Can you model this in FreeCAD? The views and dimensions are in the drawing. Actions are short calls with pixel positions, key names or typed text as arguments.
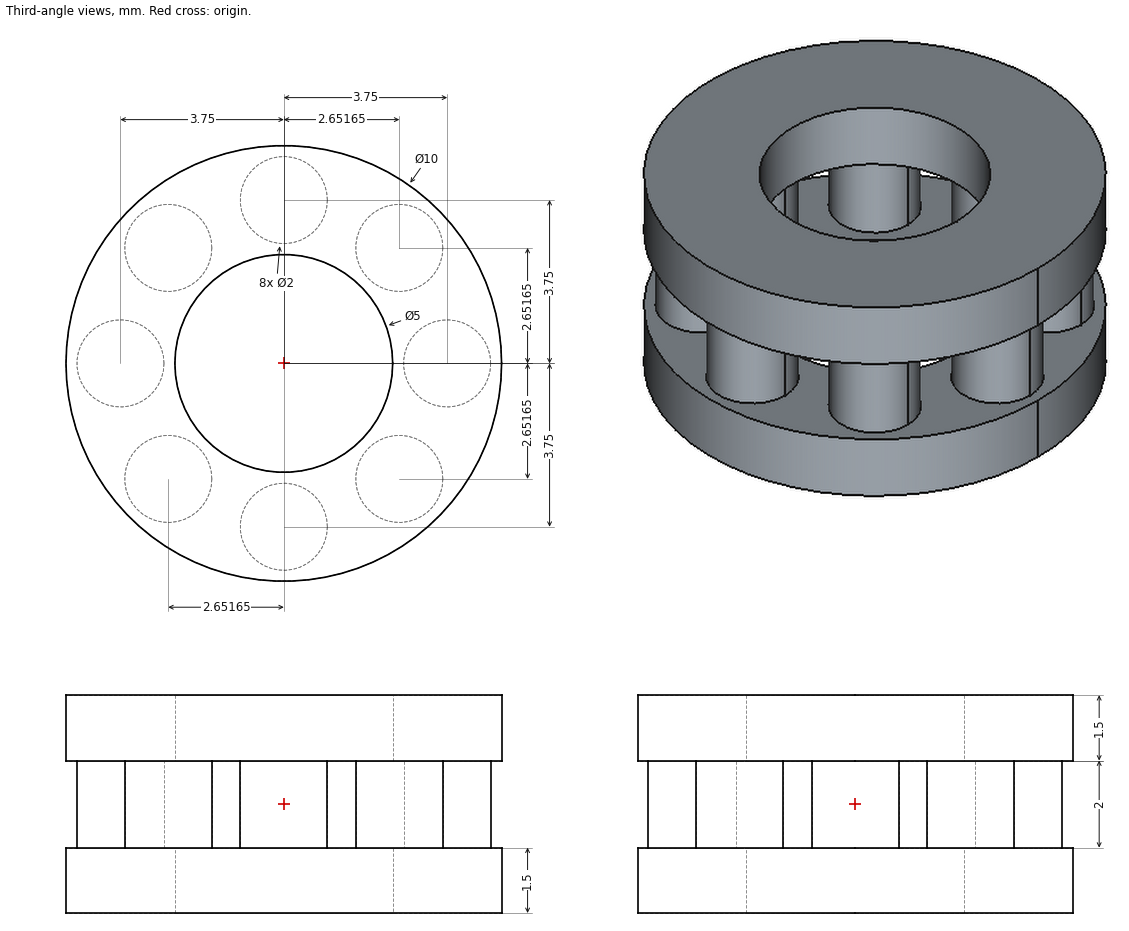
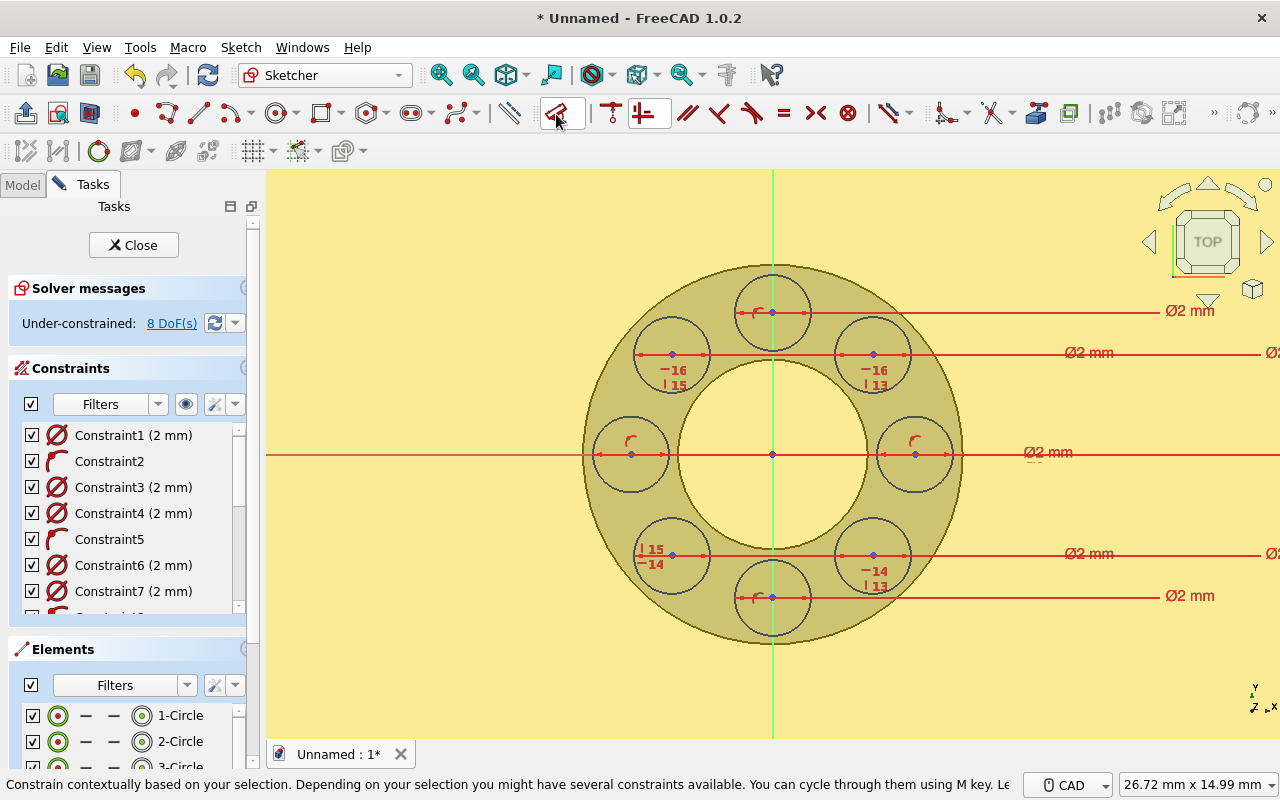
click(773, 313)
click(807, 384)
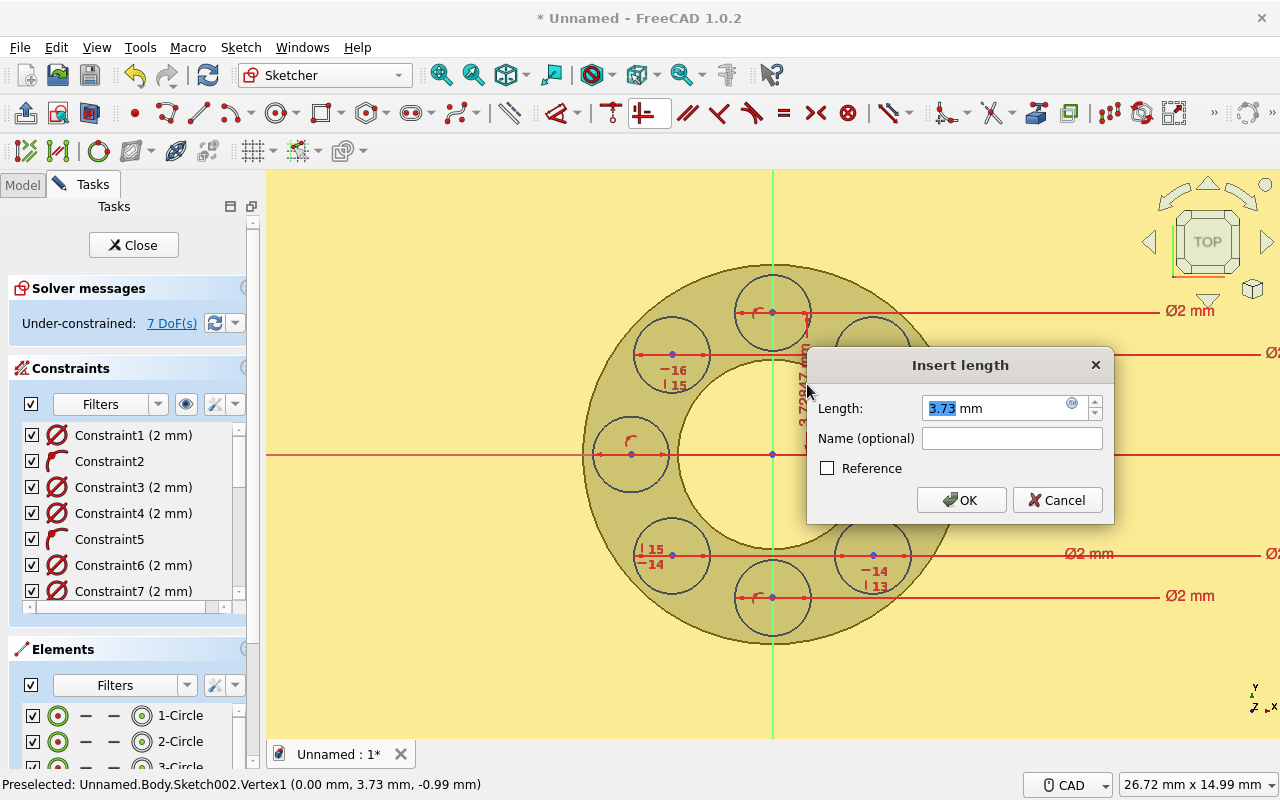
text(3.75)
key(Return)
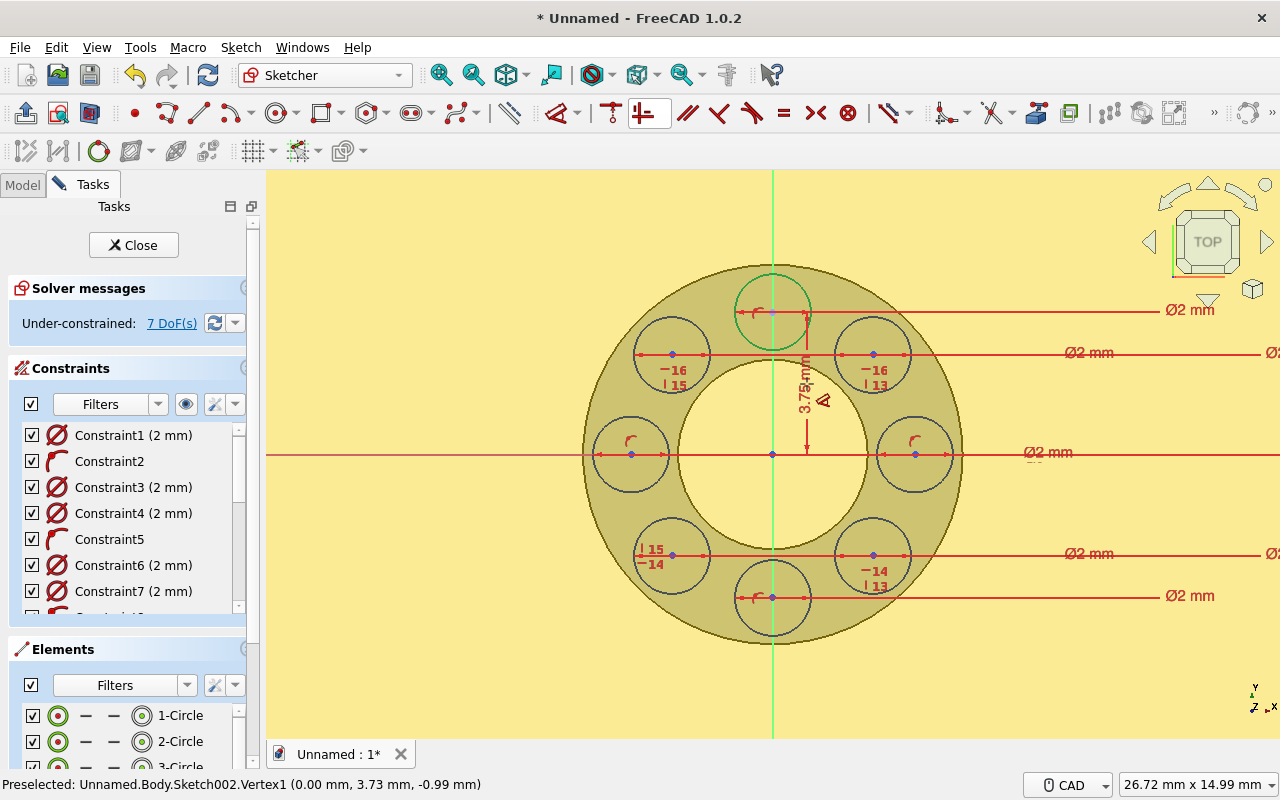
click(915, 454)
click(844, 488)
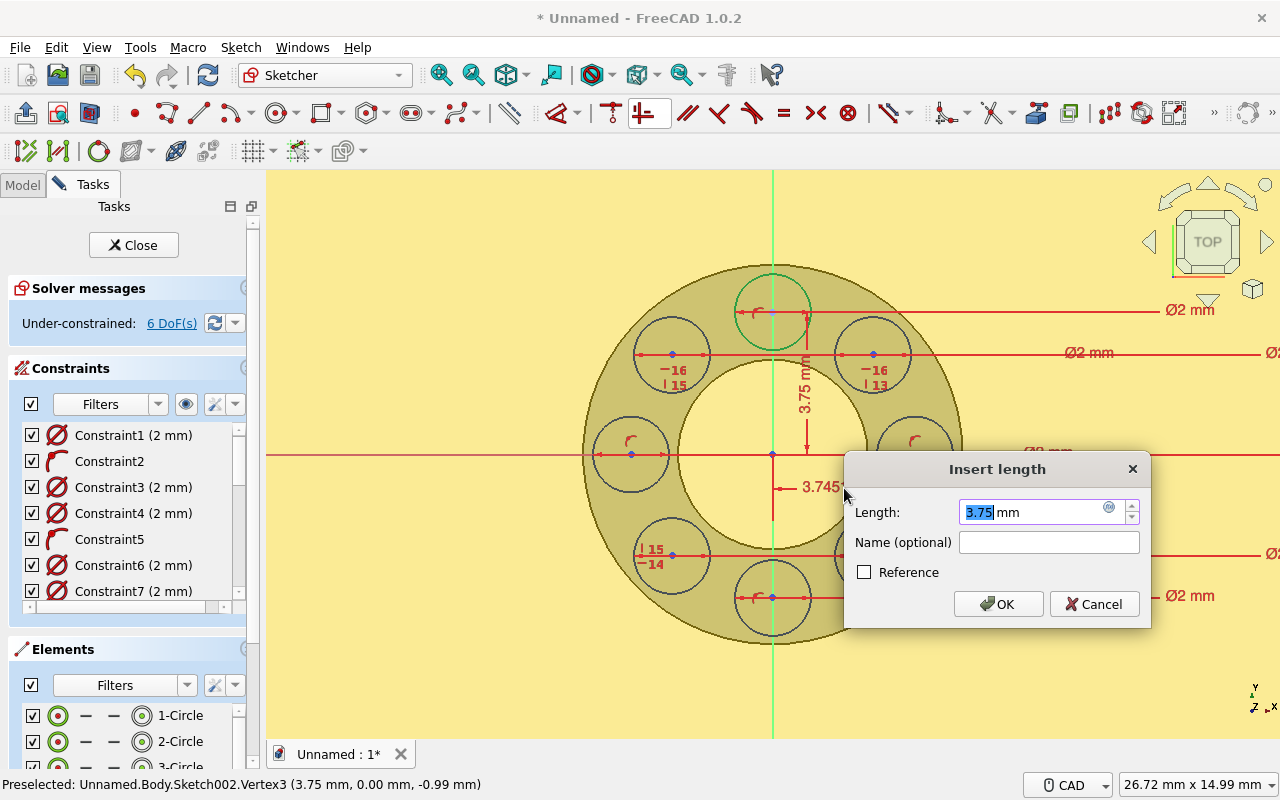
text(3.75)
key(Return)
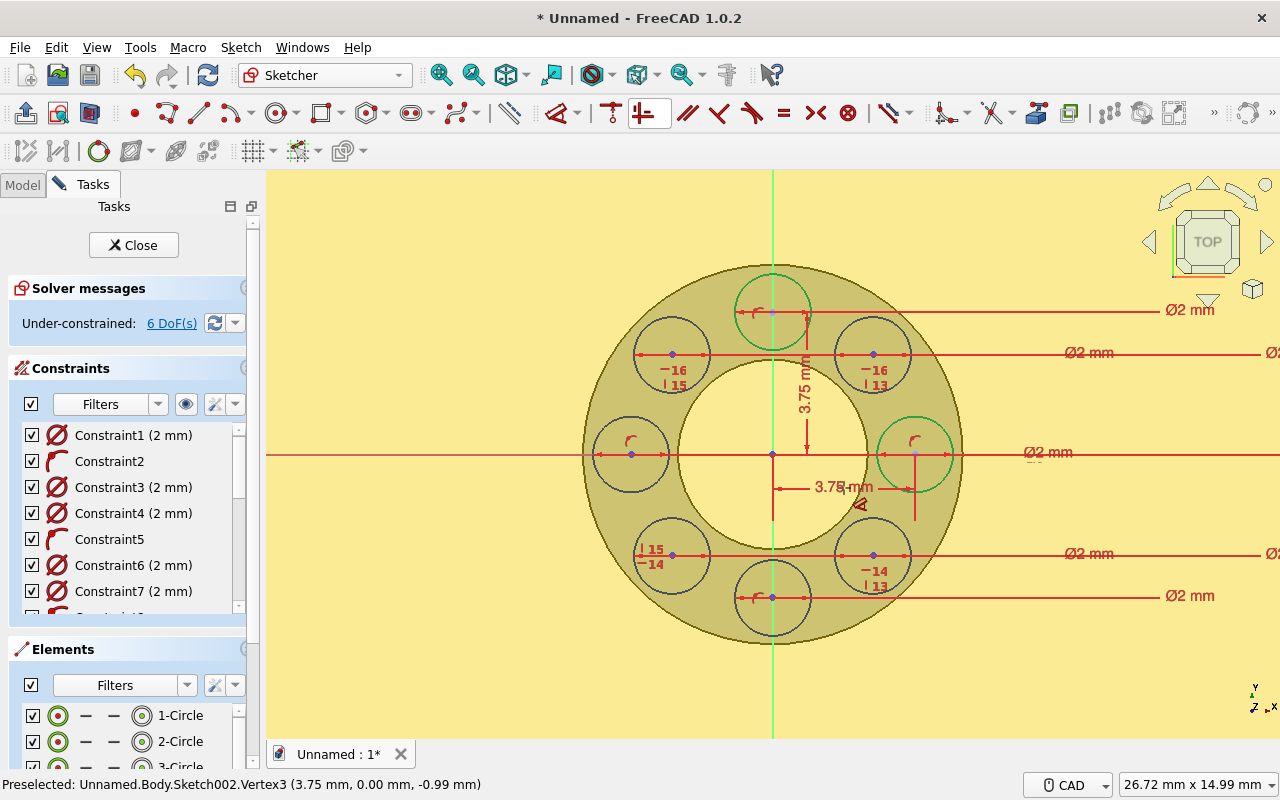
click(773, 598)
click(807, 526)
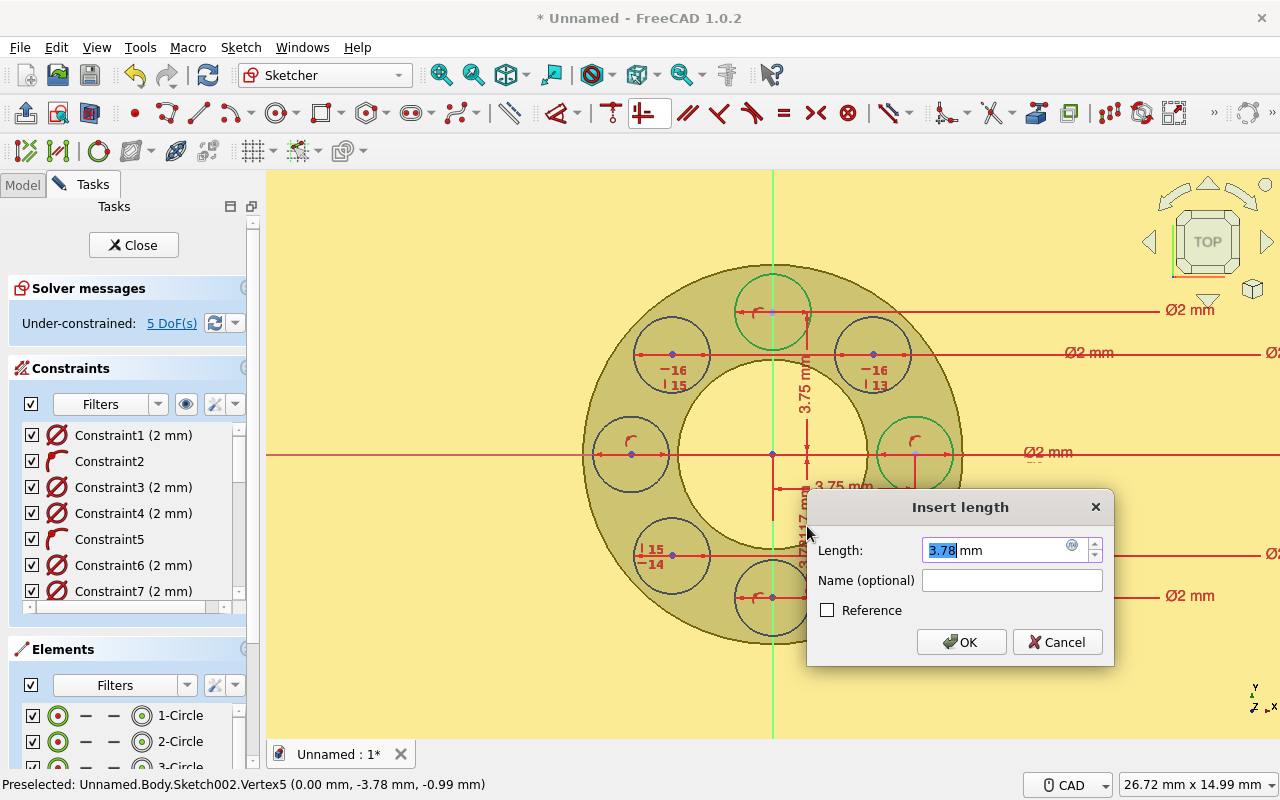
text(3.75)
key(Return)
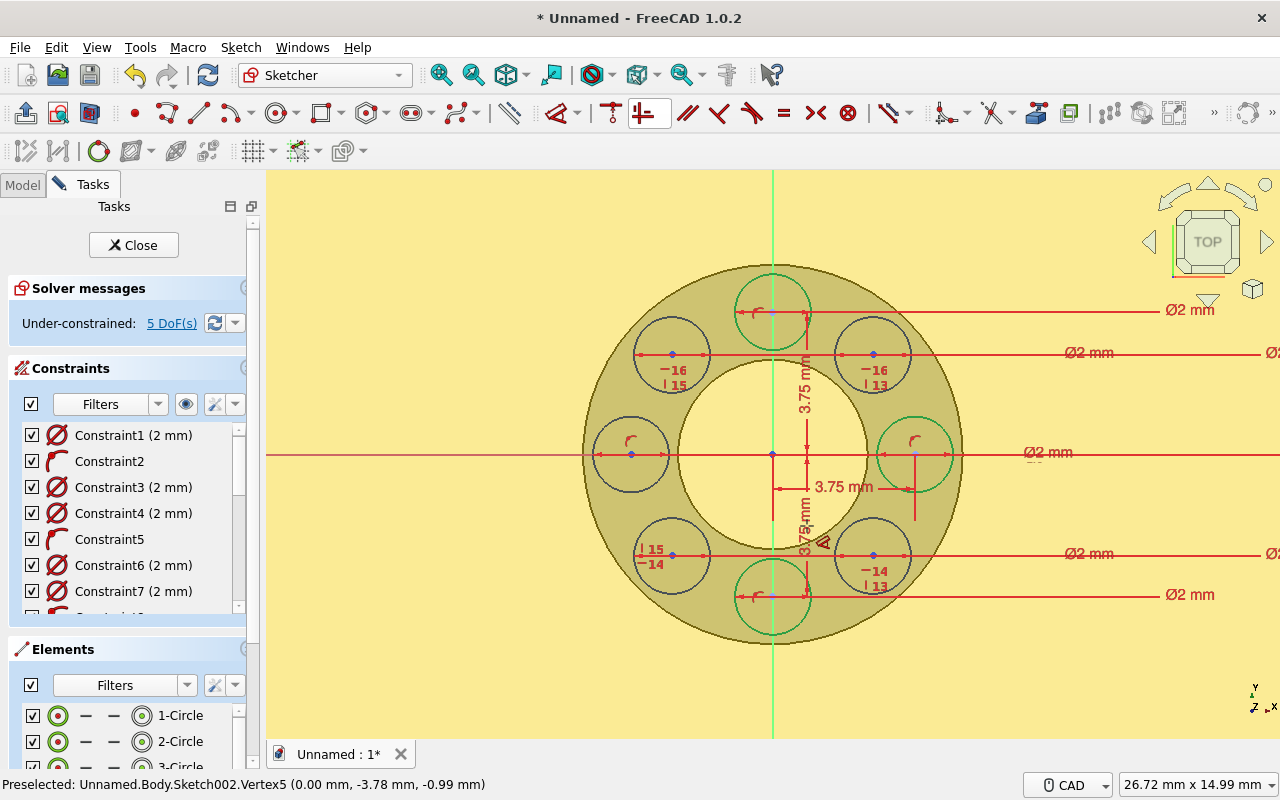
click(631, 454)
click(702, 488)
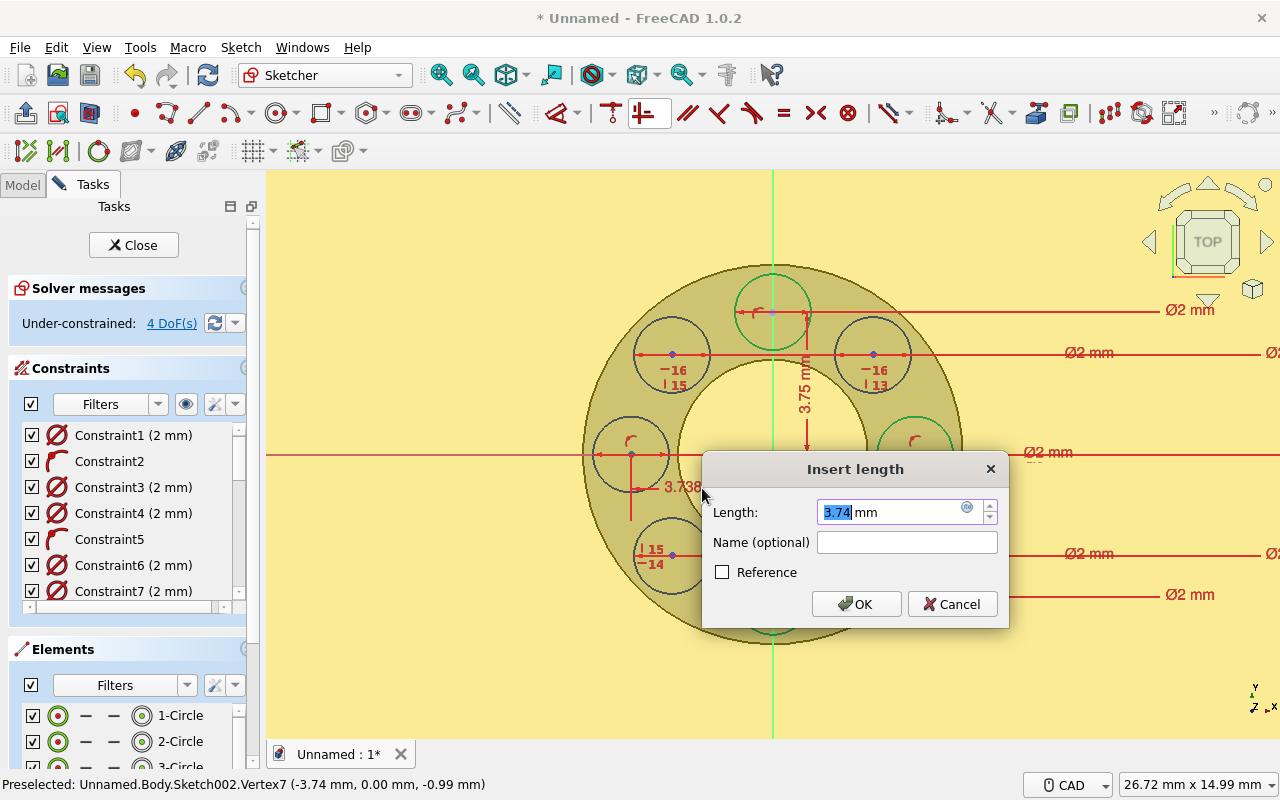
text(3.75)
key(Return)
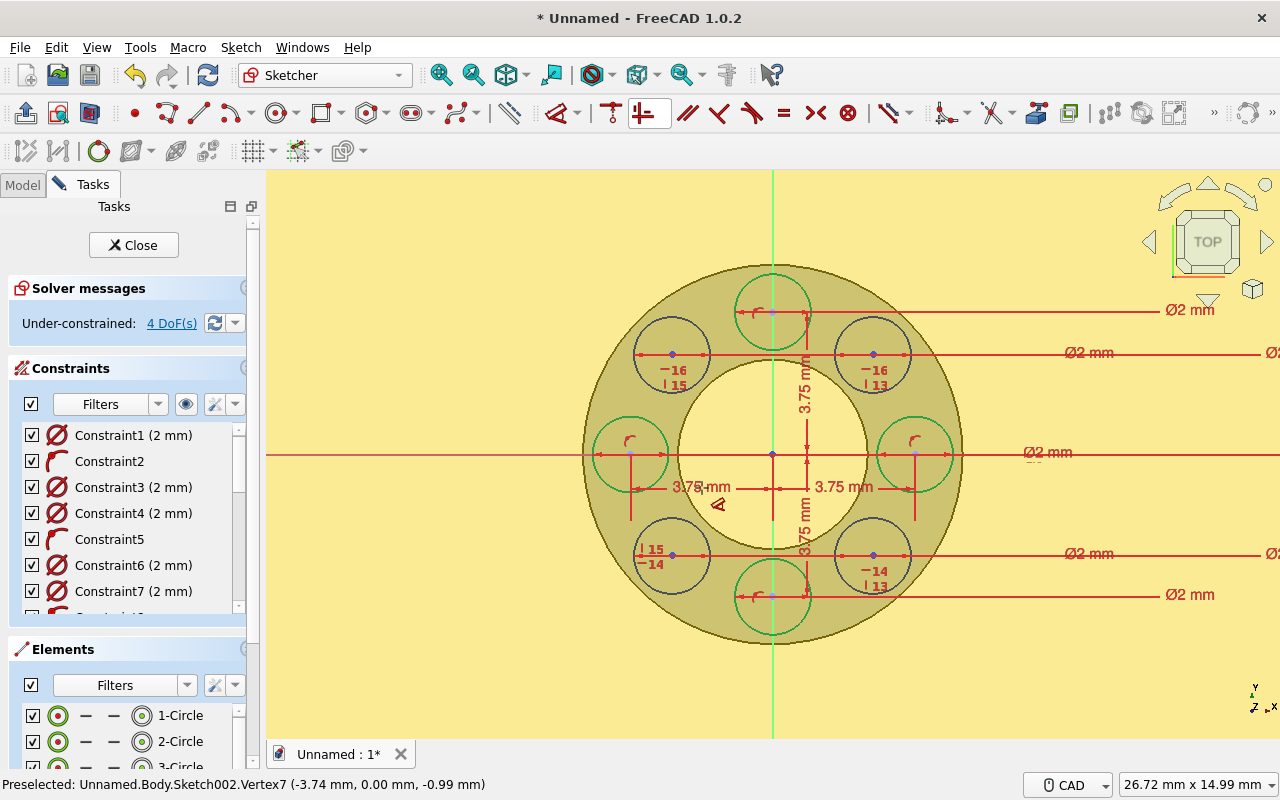
click(873, 355)
click(788, 321)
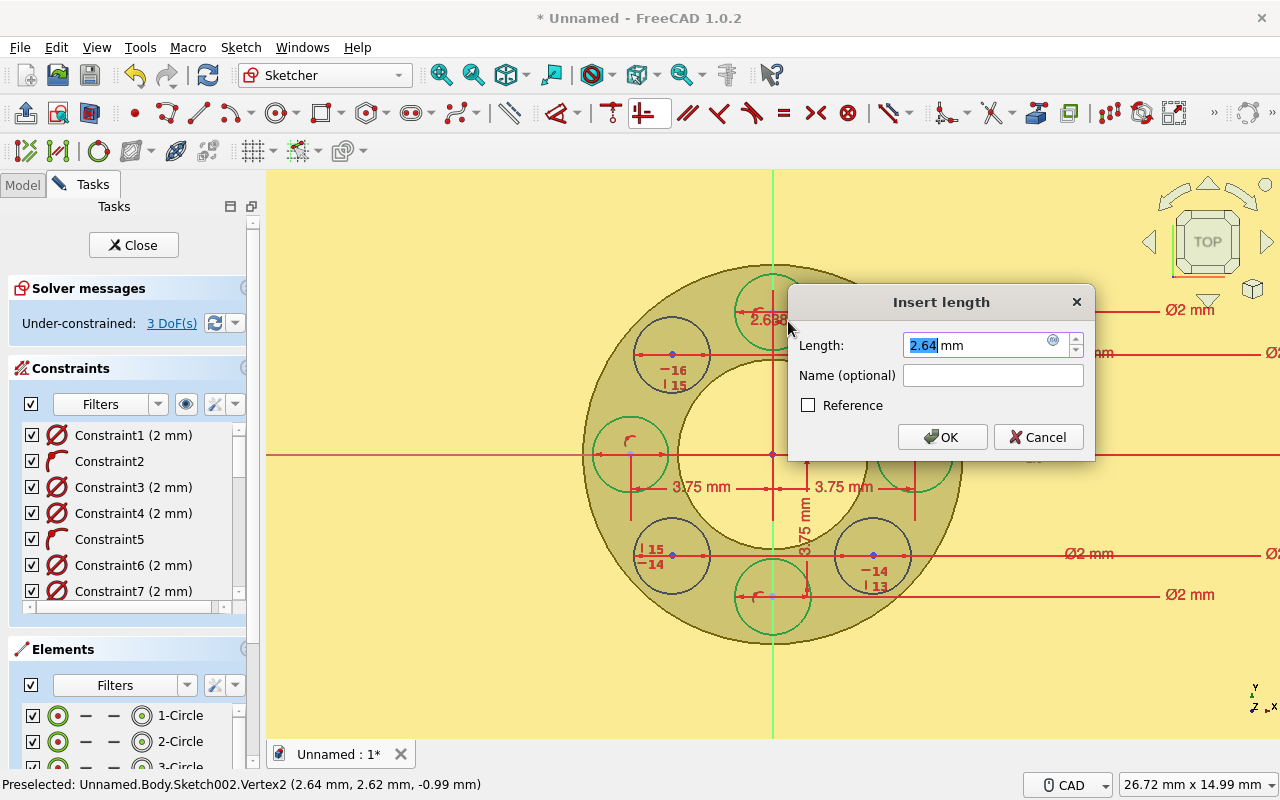
text(2.65165)
key(Return)